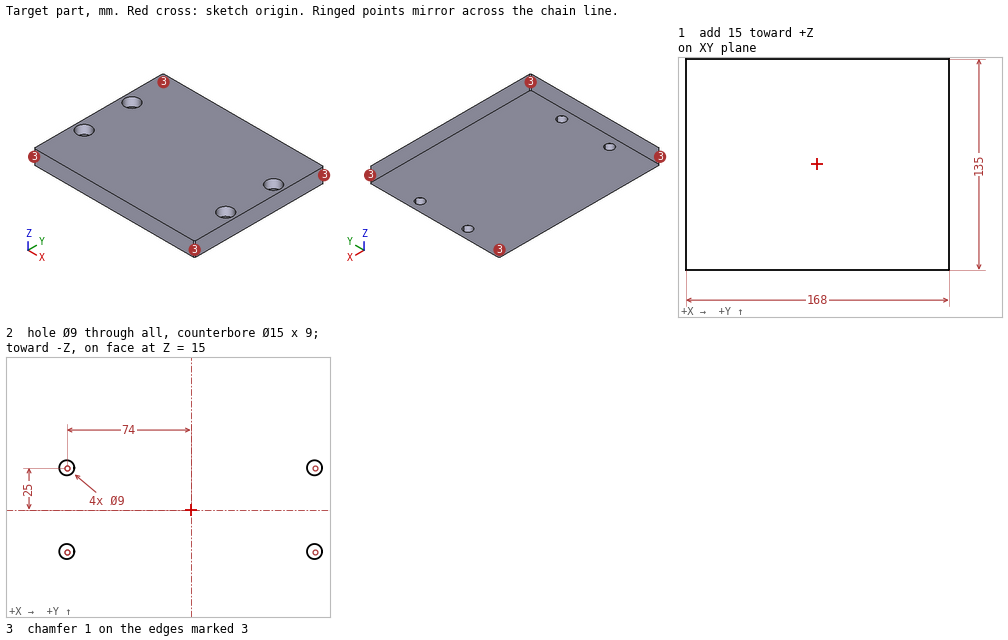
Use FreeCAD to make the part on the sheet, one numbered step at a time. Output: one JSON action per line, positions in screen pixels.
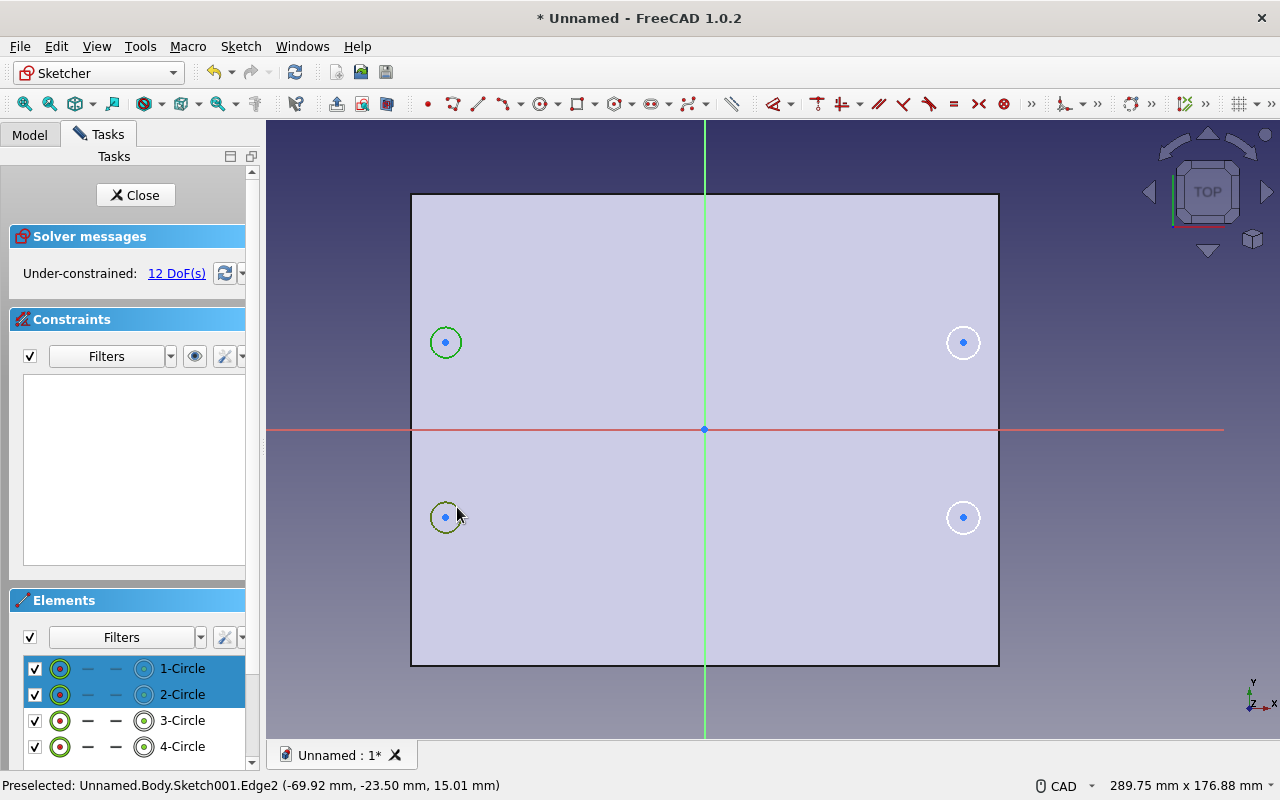
{"action": "left_click", "coordinate": [975, 506]}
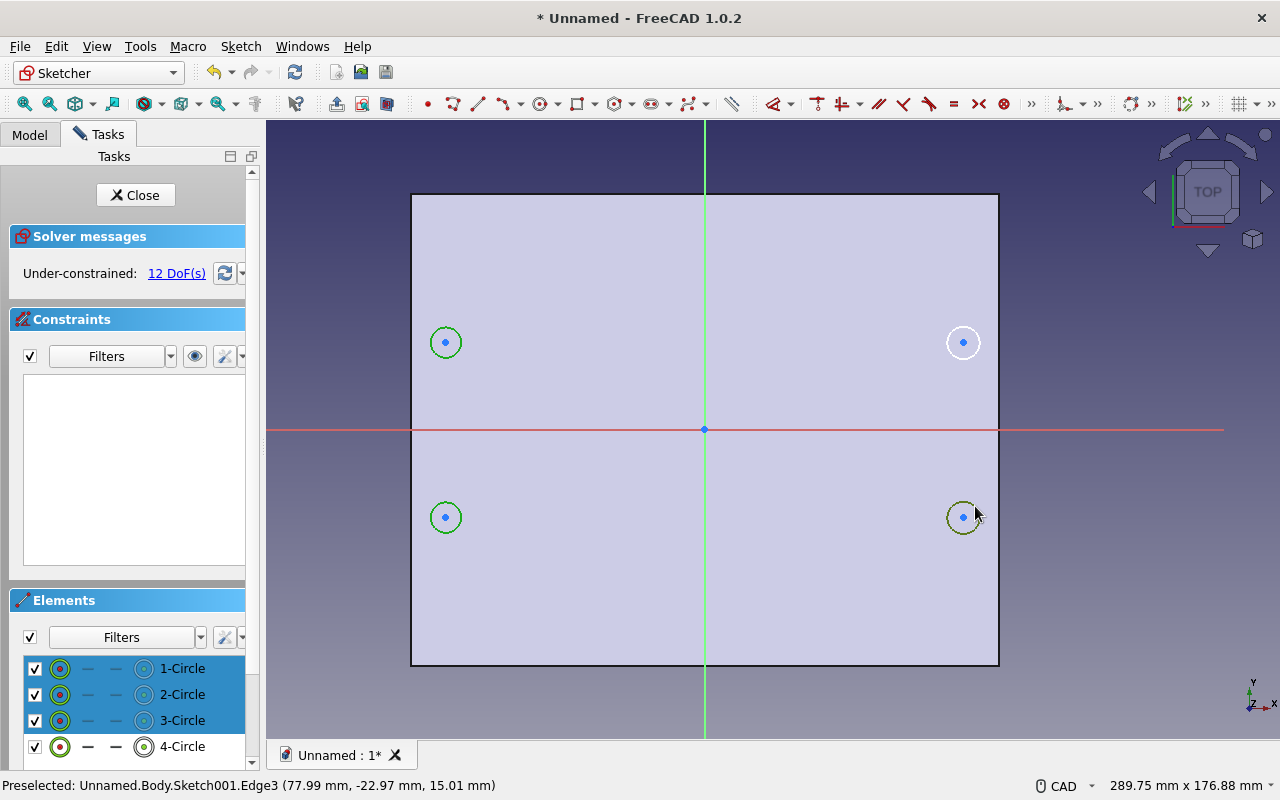
{"action": "left_click", "coordinate": [975, 331]}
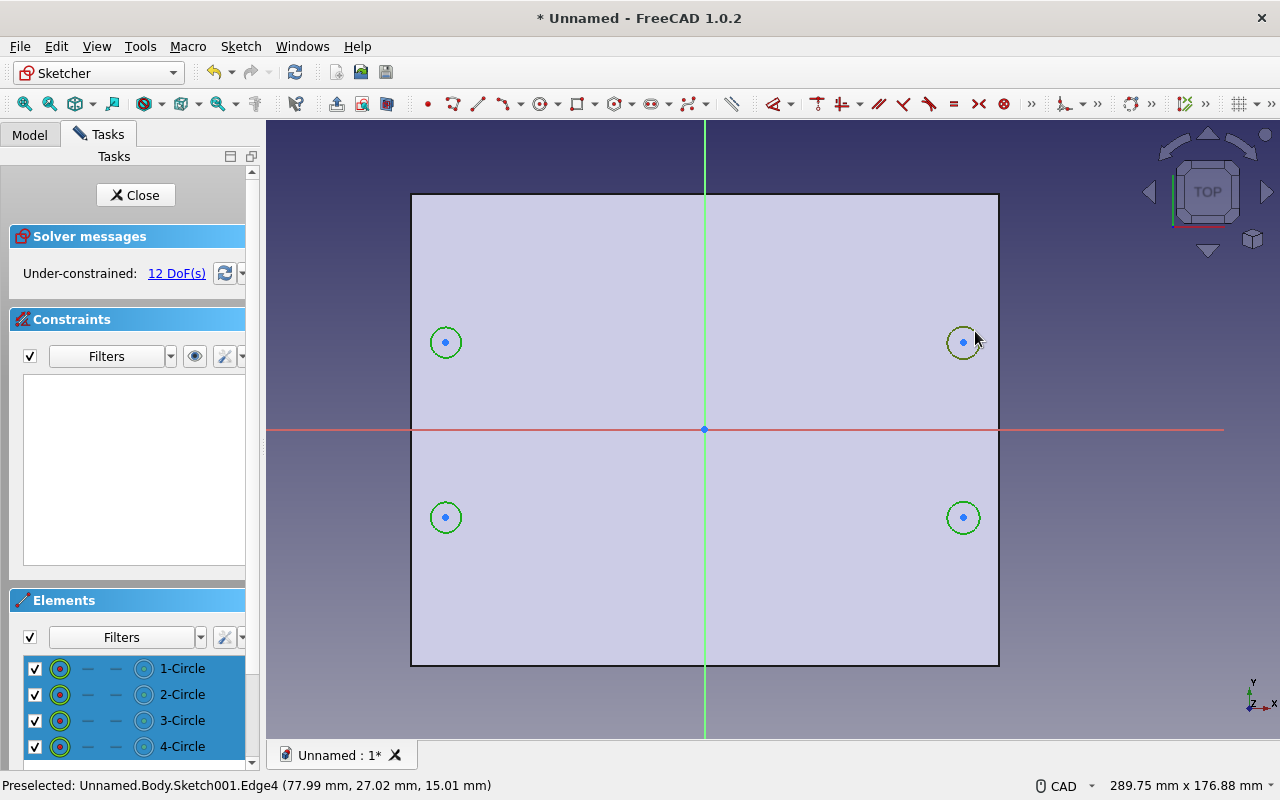
{"action": "key", "text": "e"}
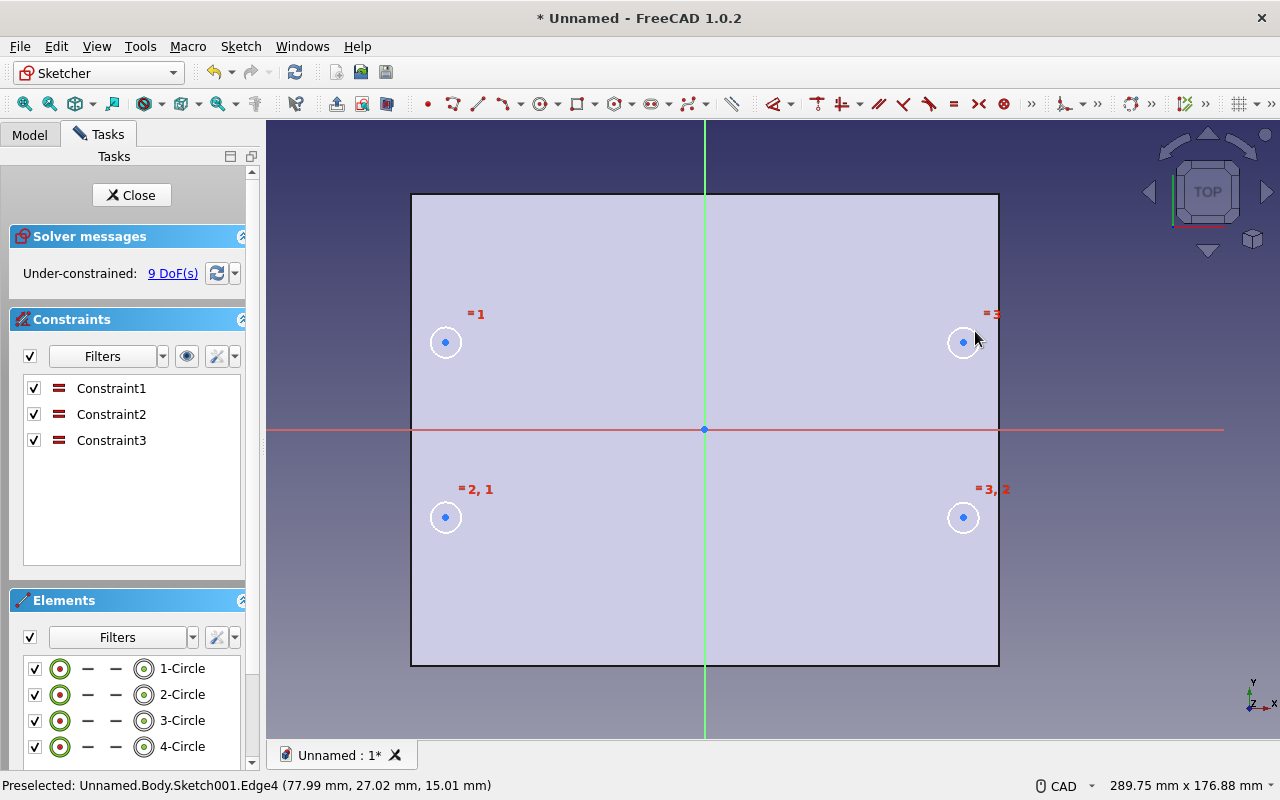
{"action": "left_click", "coordinate": [446, 343]}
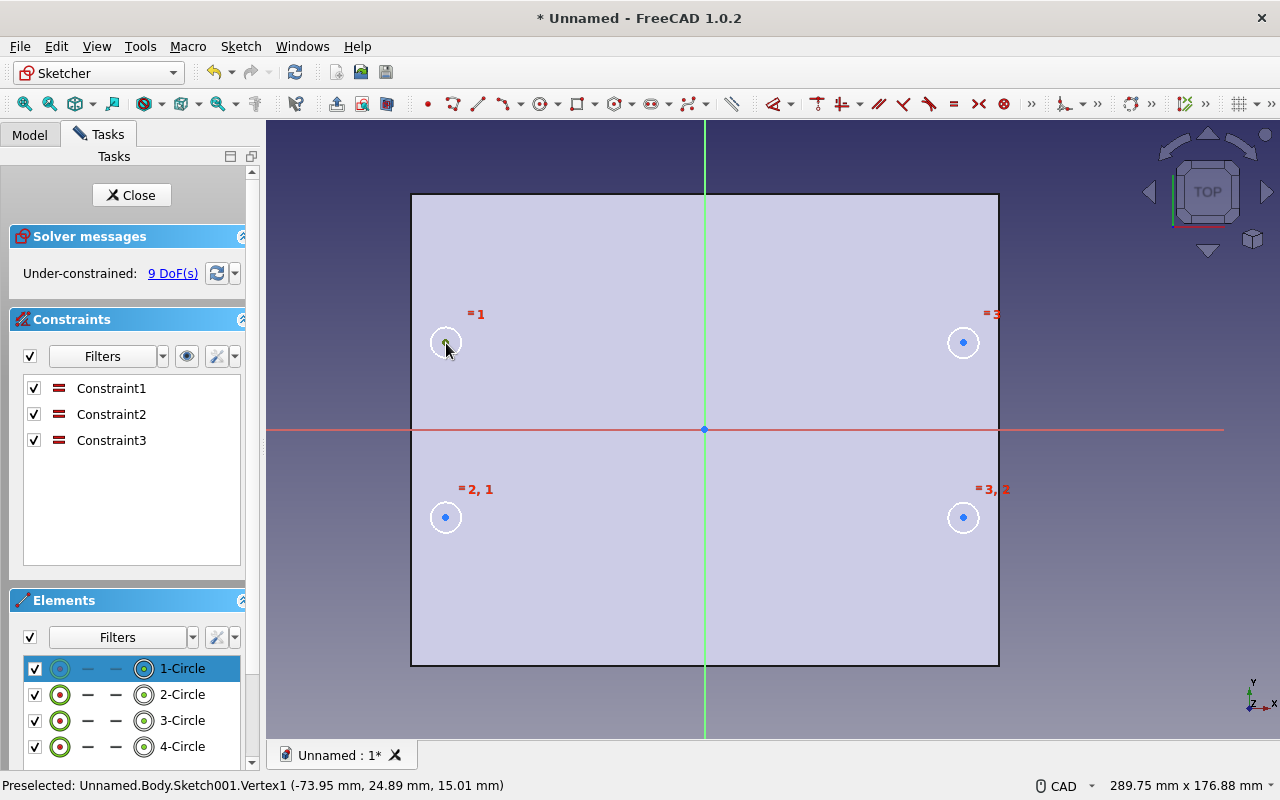
{"action": "left_click", "coordinate": [446, 518]}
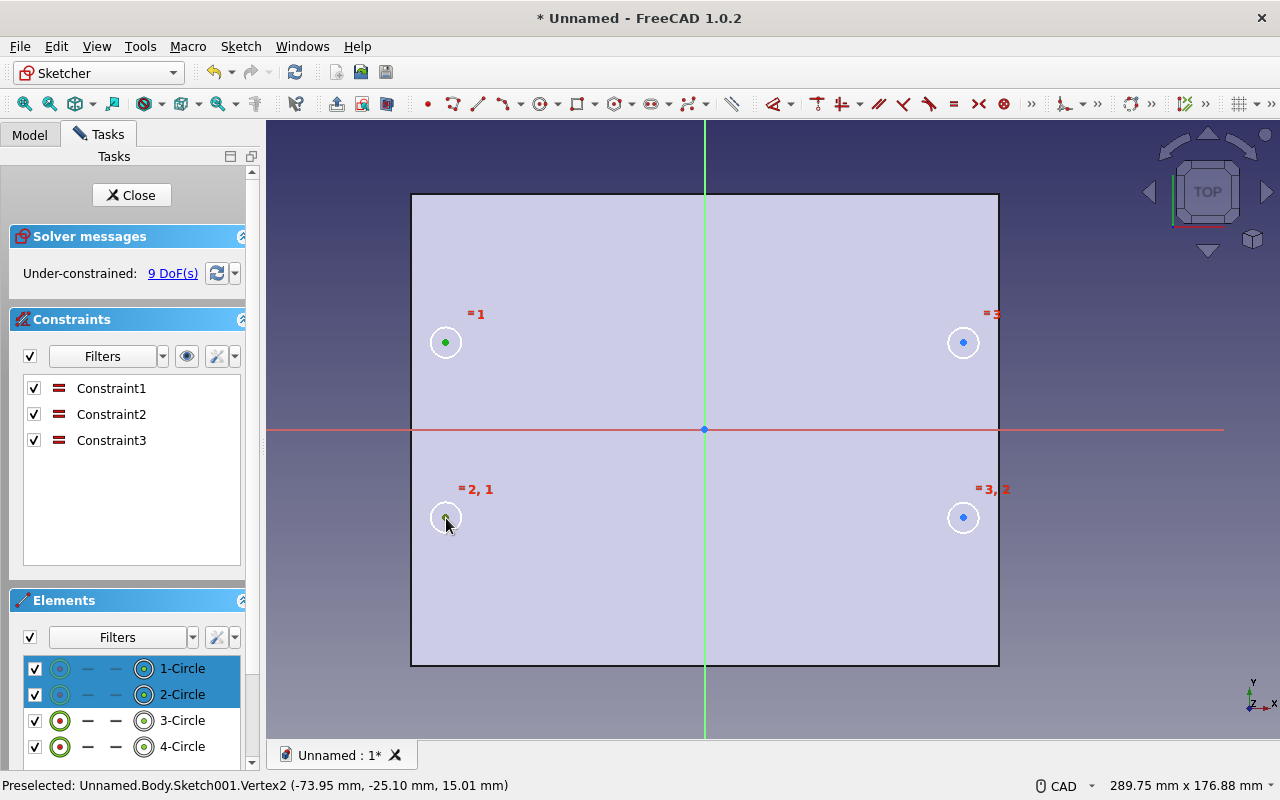
{"action": "left_click", "coordinate": [353, 430]}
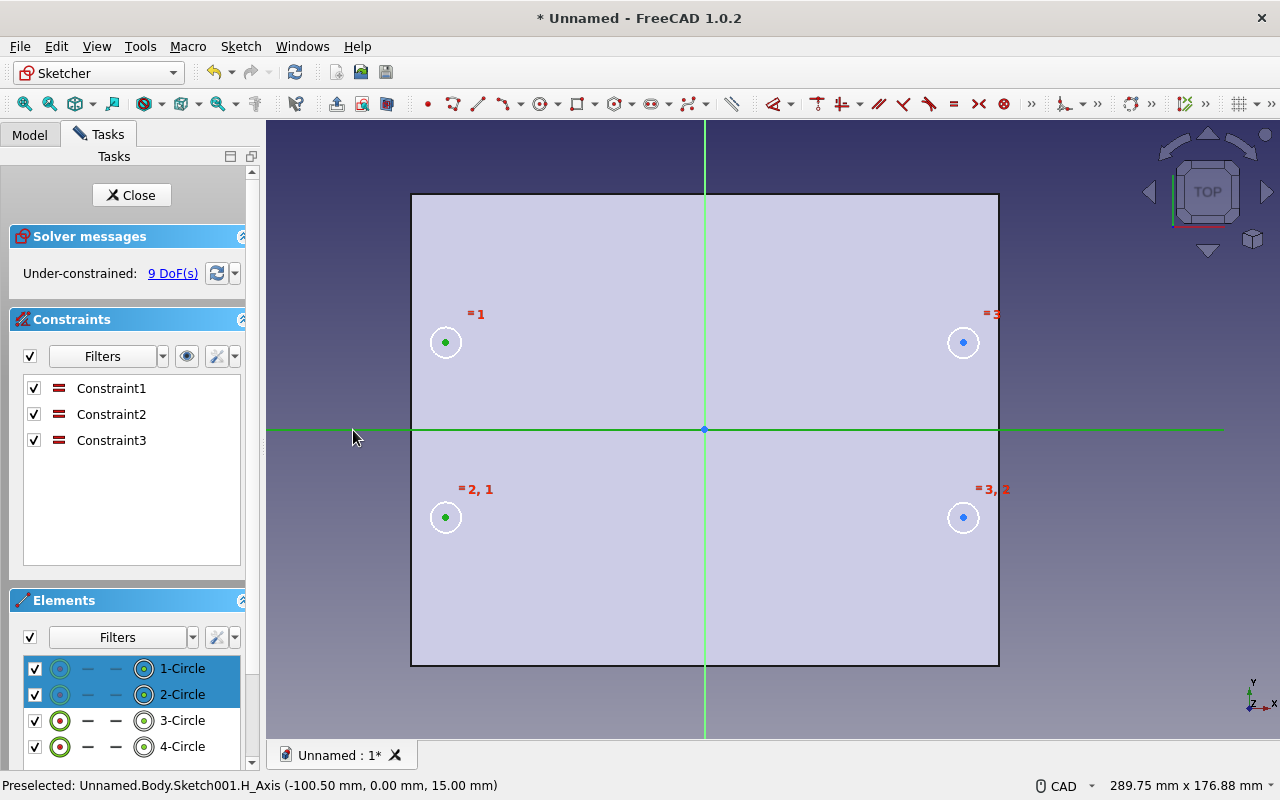
{"action": "left_click", "coordinate": [979, 104]}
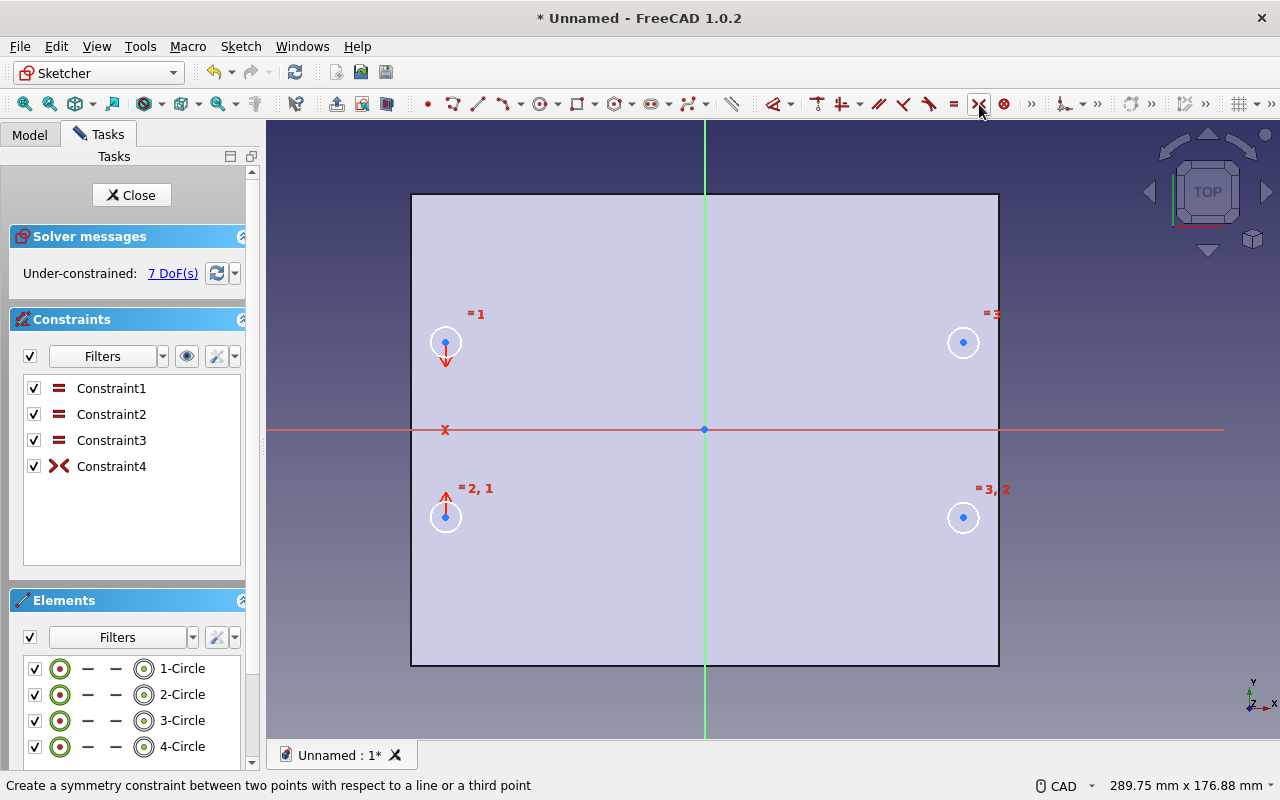
{"action": "left_click", "coordinate": [446, 517]}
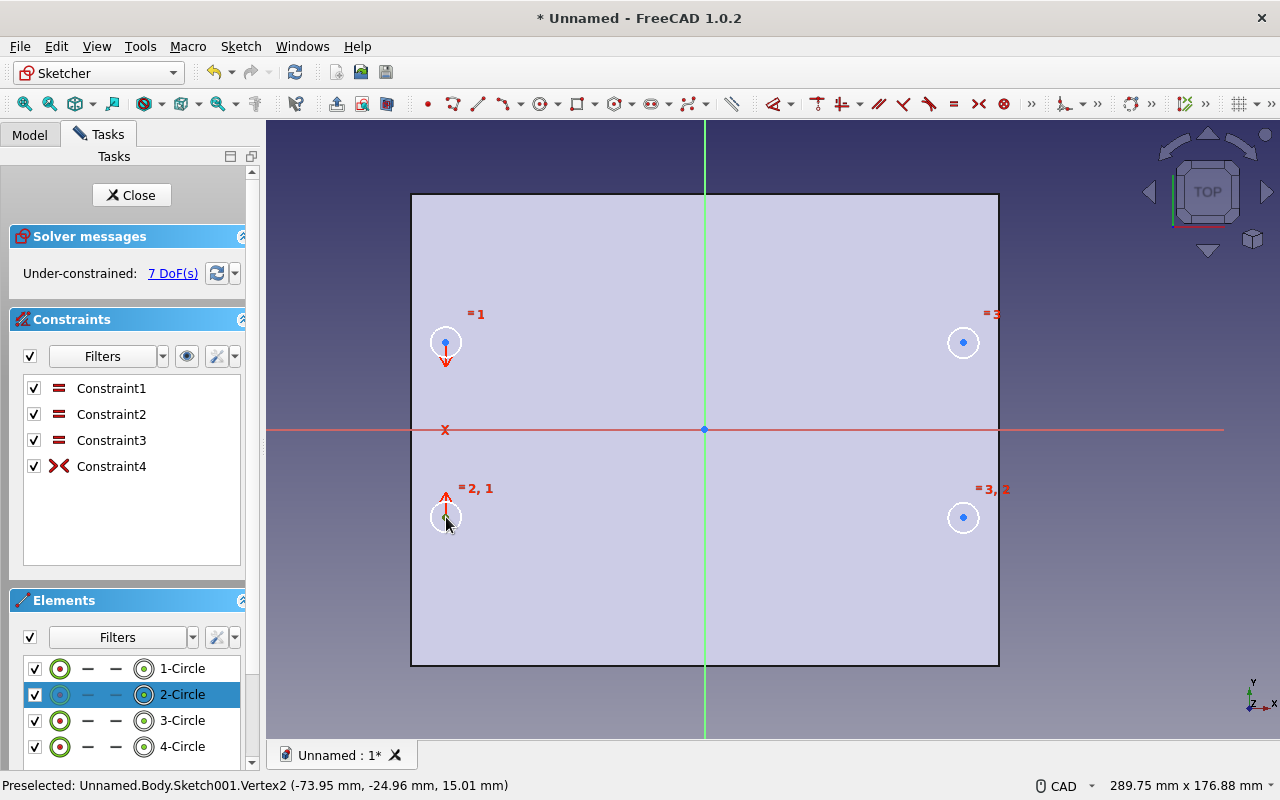
{"action": "left_click", "coordinate": [964, 518]}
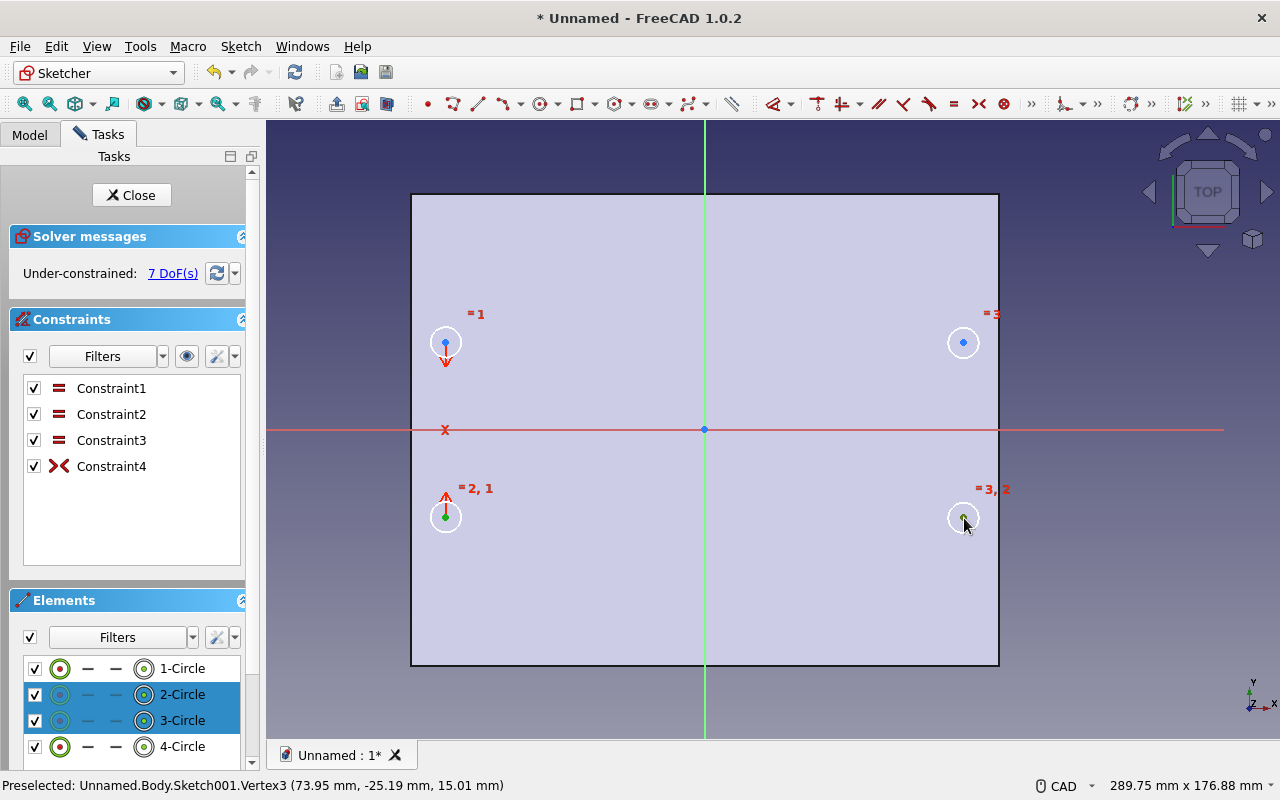
{"action": "left_click", "coordinate": [705, 671]}